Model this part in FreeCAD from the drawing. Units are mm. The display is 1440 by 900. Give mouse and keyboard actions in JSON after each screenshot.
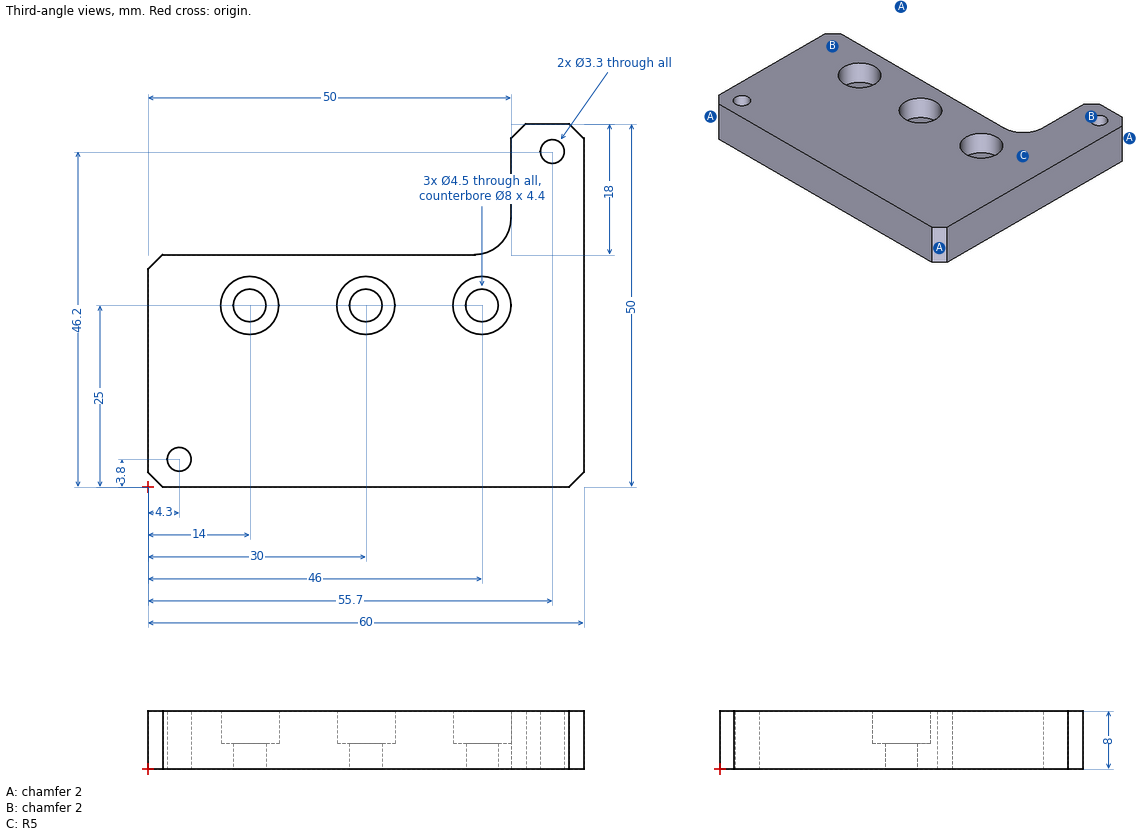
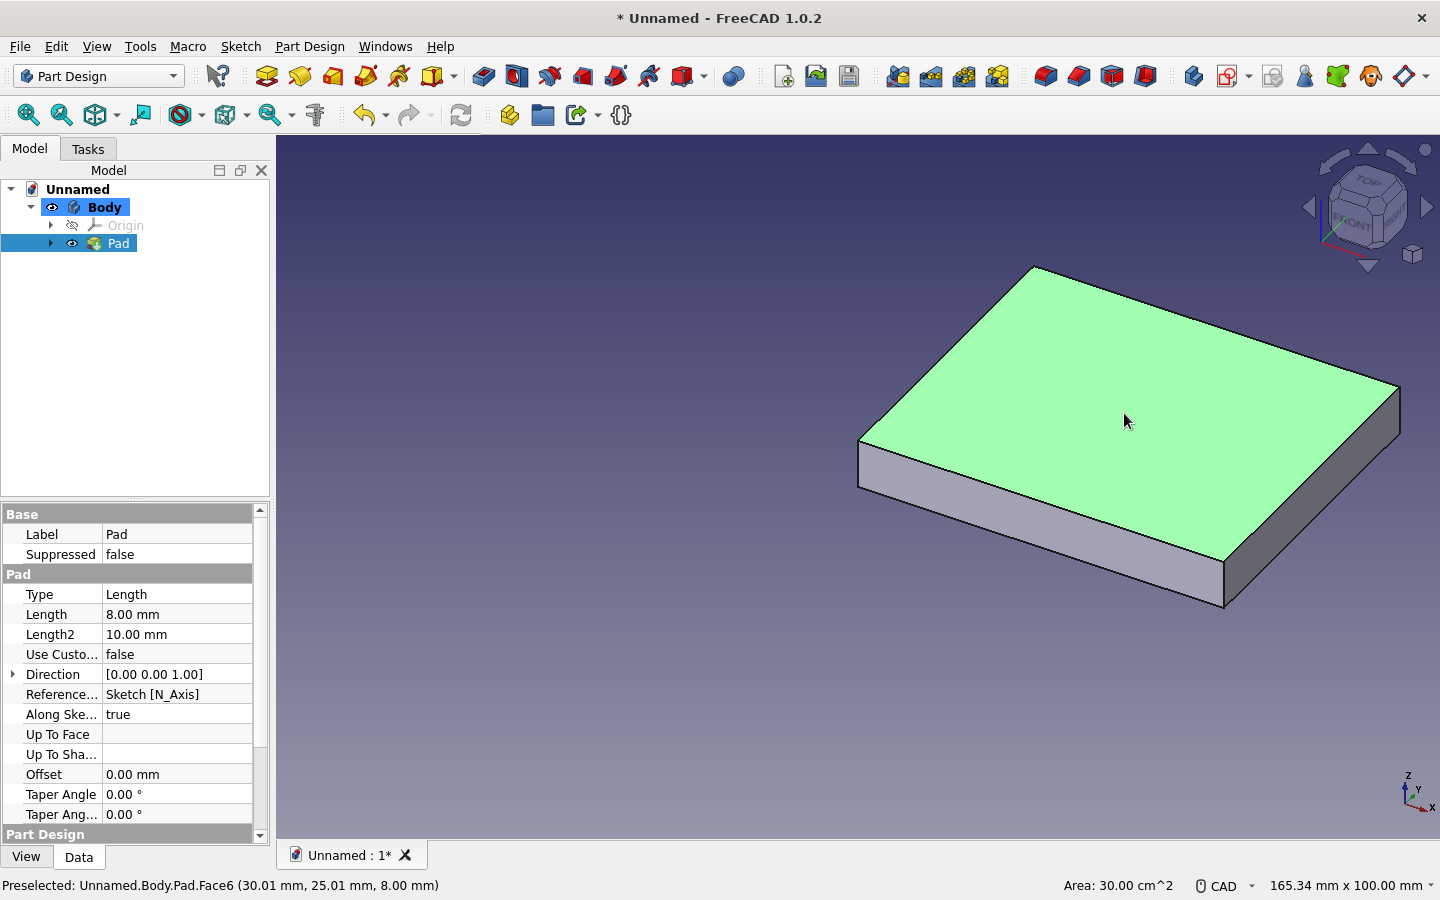
{"action": "left_click", "coordinate": [1226, 76]}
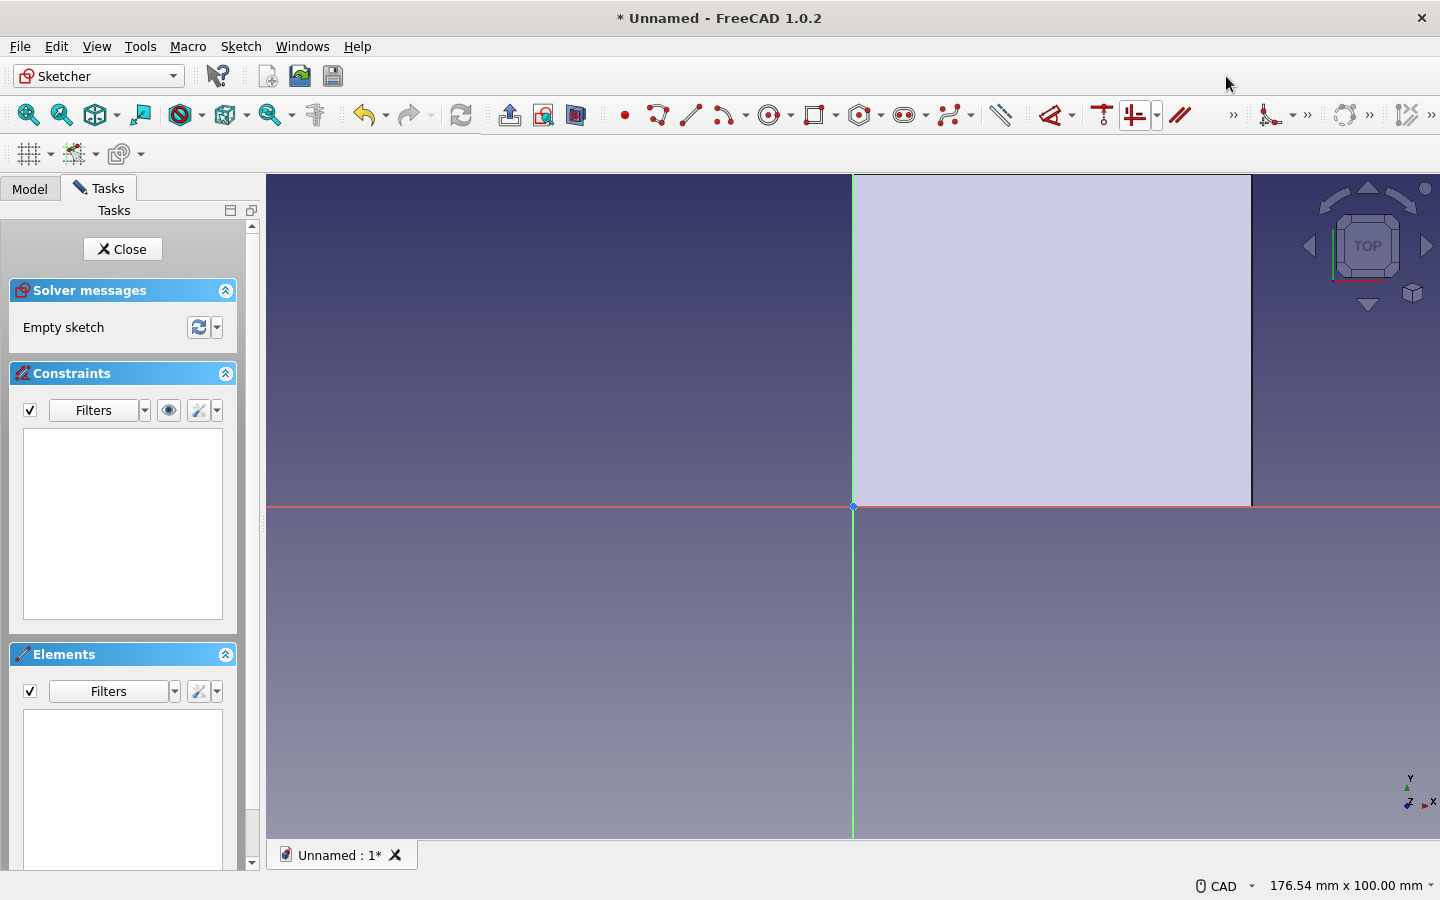
{"action": "scroll", "coordinate": [1200, 342], "scroll_direction": "up", "scroll_amount": 4}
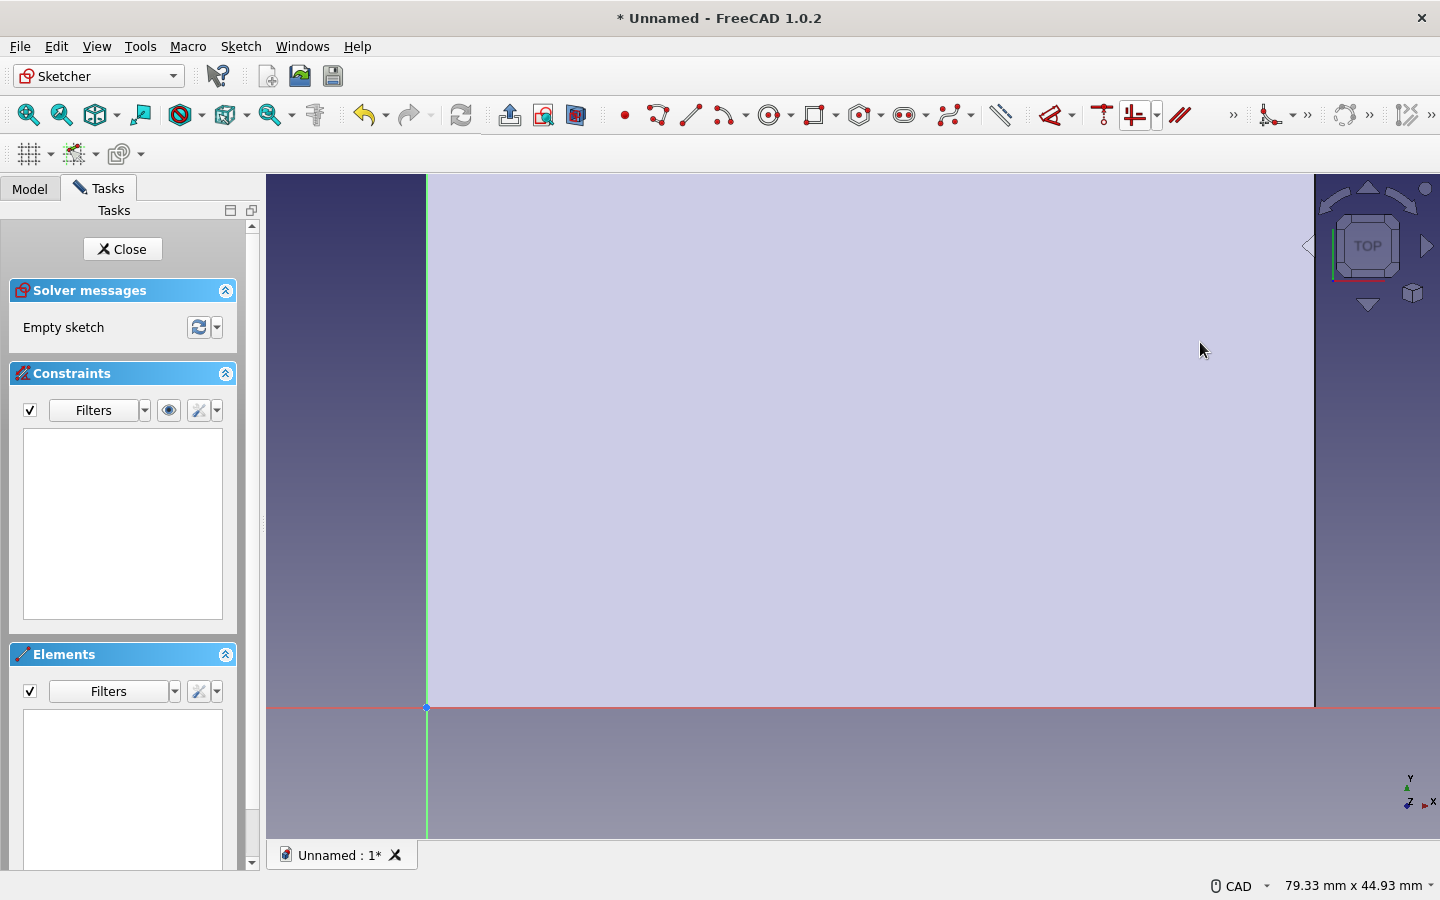
{"action": "left_click", "coordinate": [768, 116]}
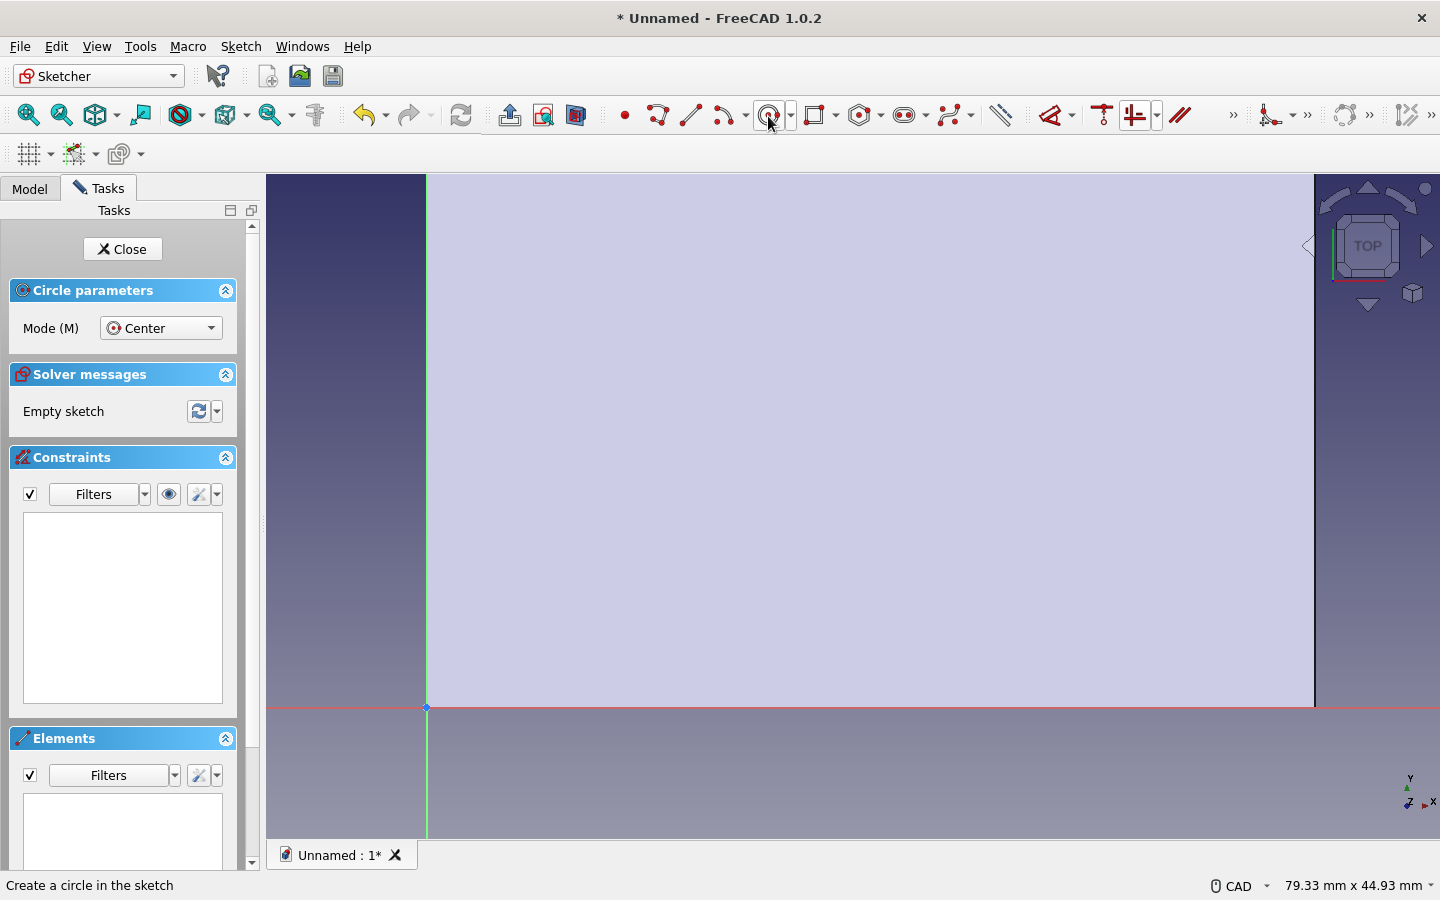
{"action": "left_click", "coordinate": [1108, 338]}
{"action": "mouse_move", "coordinate": [1131, 314]}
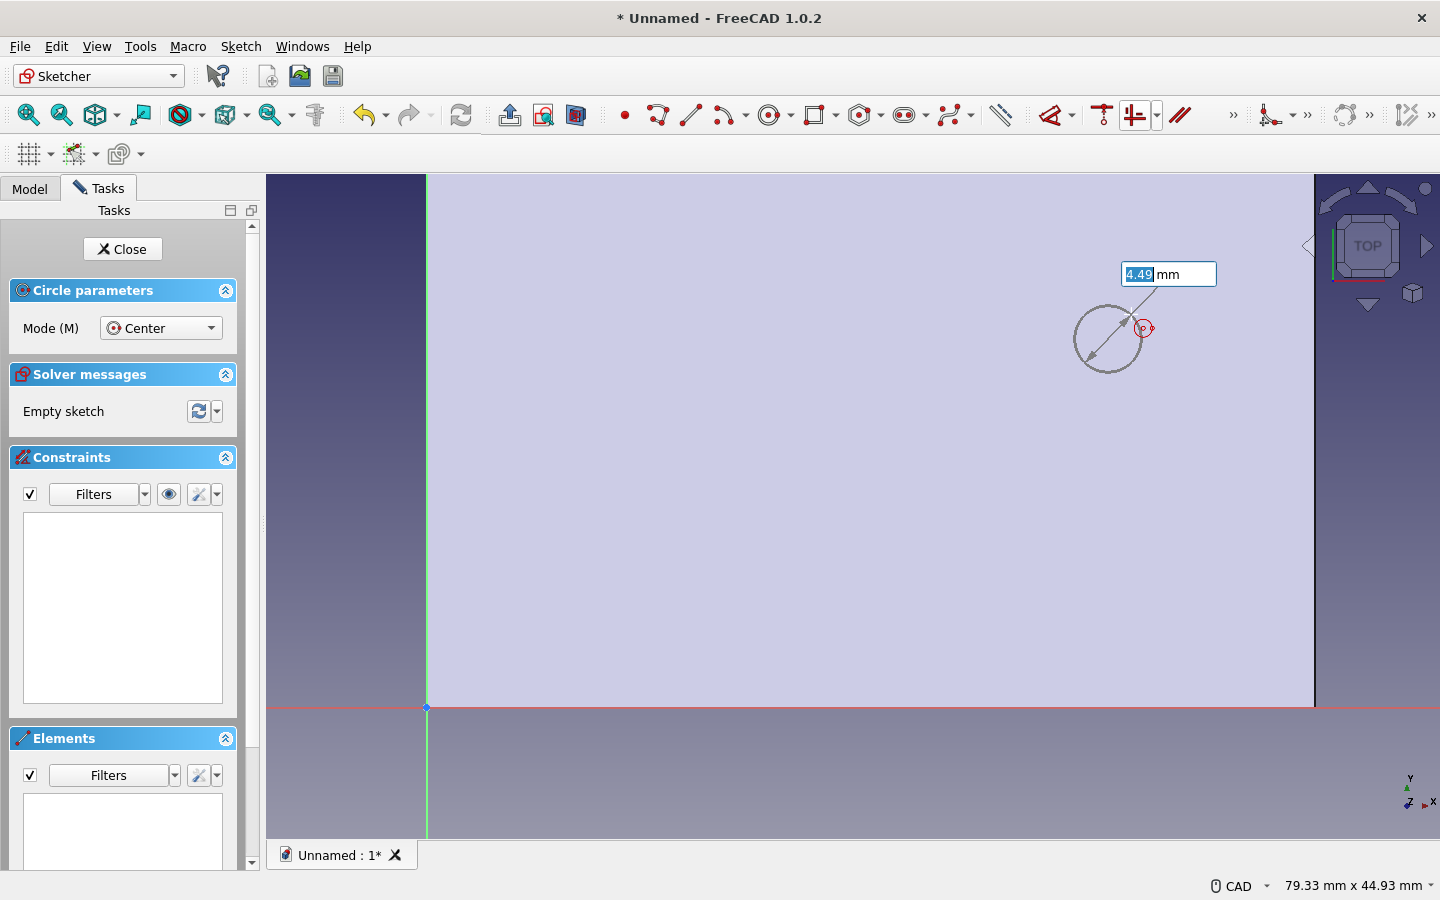
{"action": "type", "text": "4.5"}
{"action": "key", "text": "Return"}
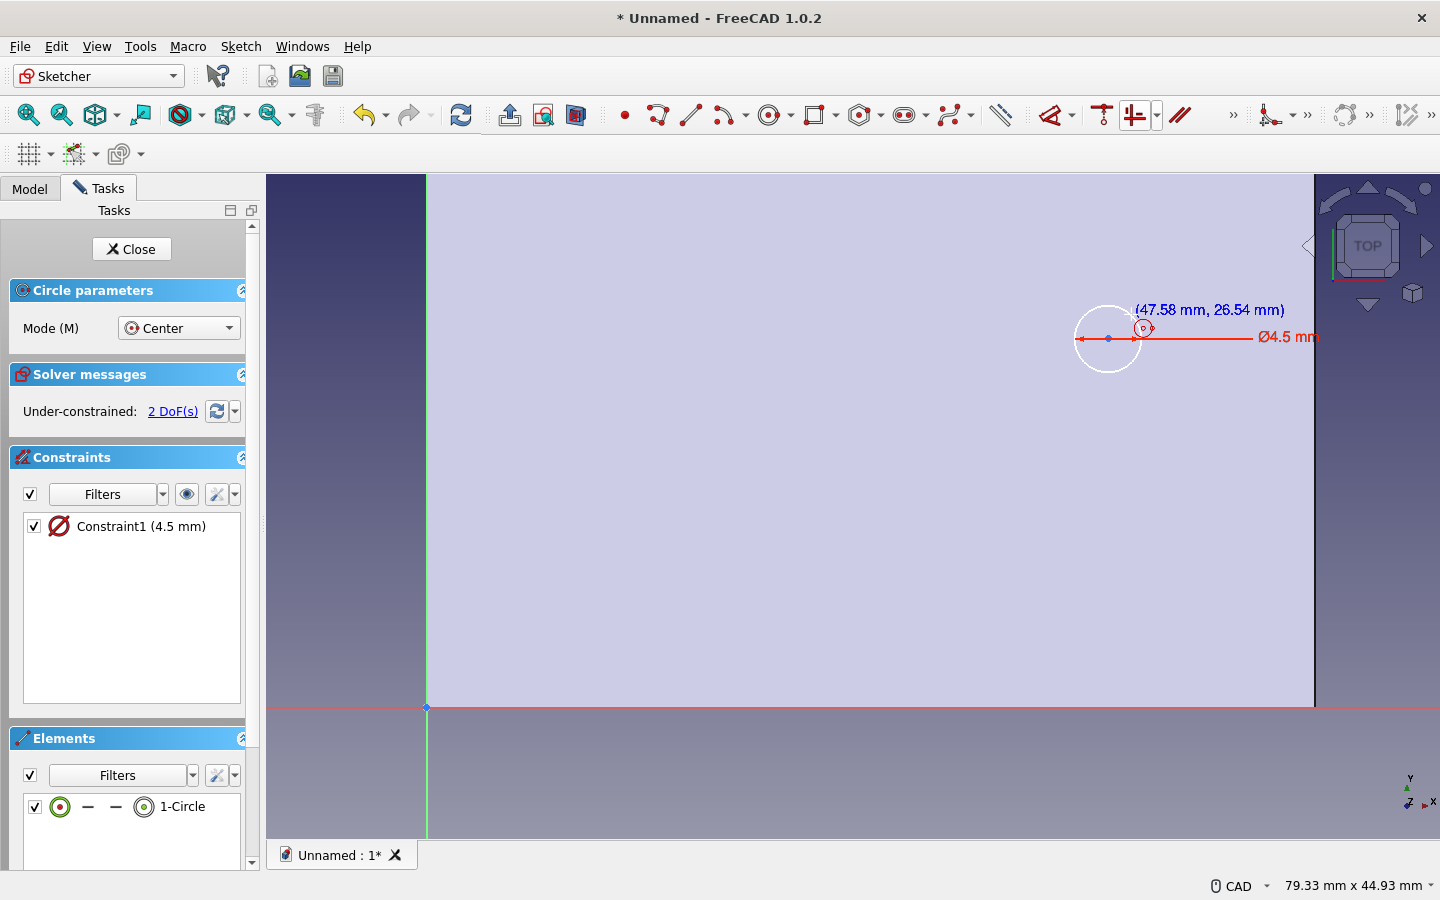
{"action": "left_click", "coordinate": [871, 338]}
{"action": "mouse_move", "coordinate": [894, 314]}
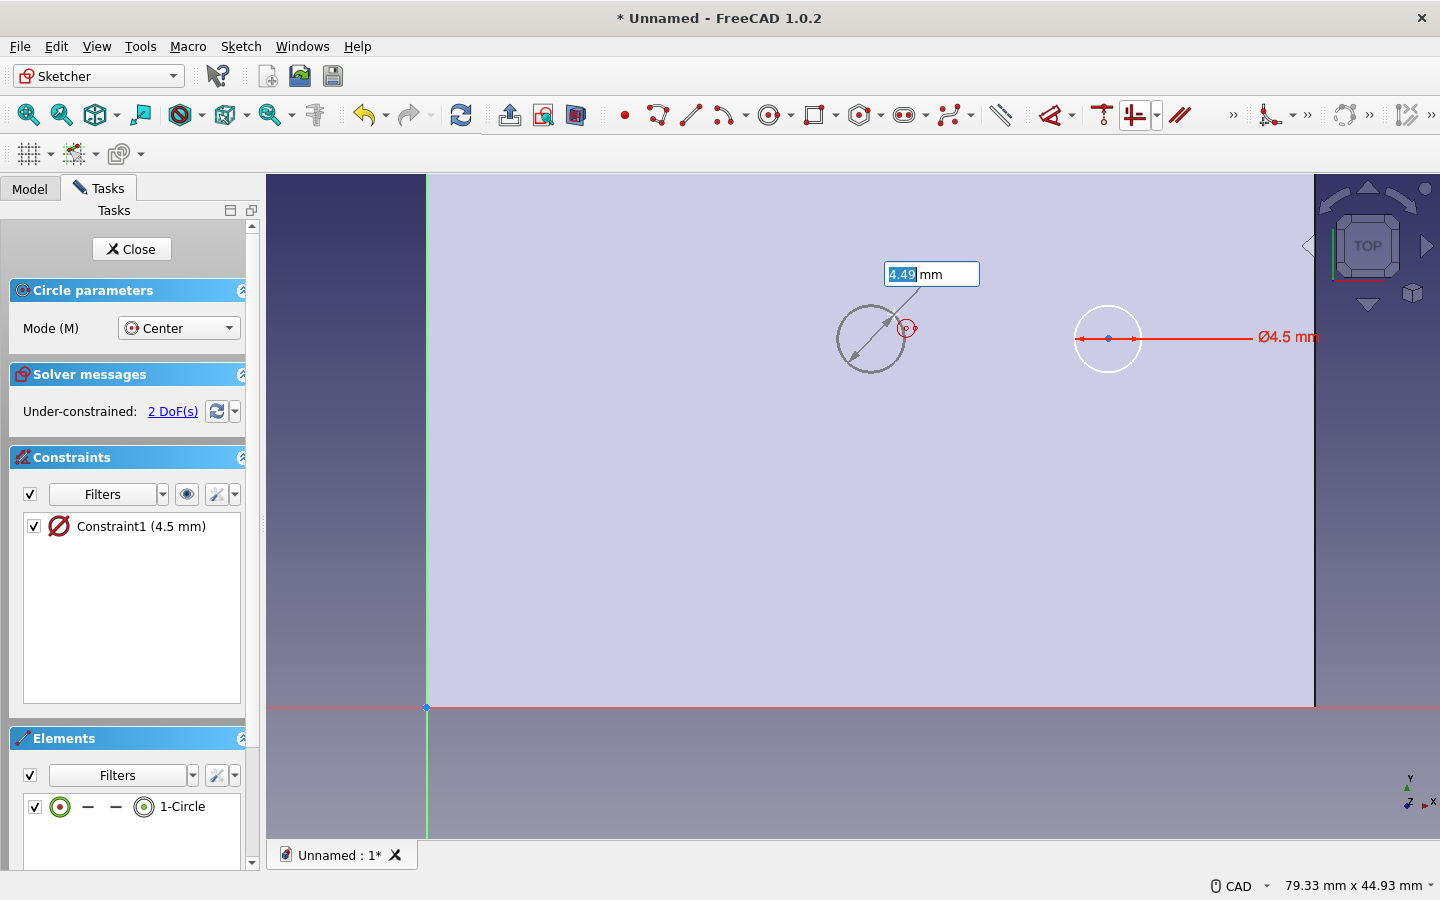
{"action": "type", "text": "4.5"}
{"action": "key", "text": "Return"}